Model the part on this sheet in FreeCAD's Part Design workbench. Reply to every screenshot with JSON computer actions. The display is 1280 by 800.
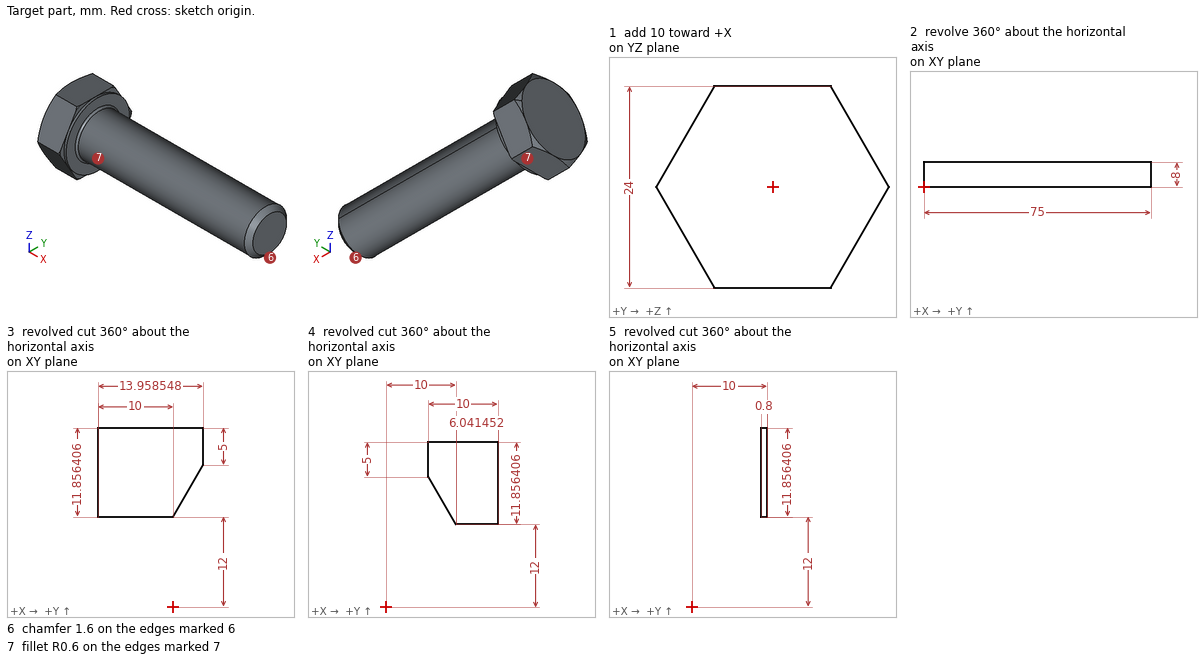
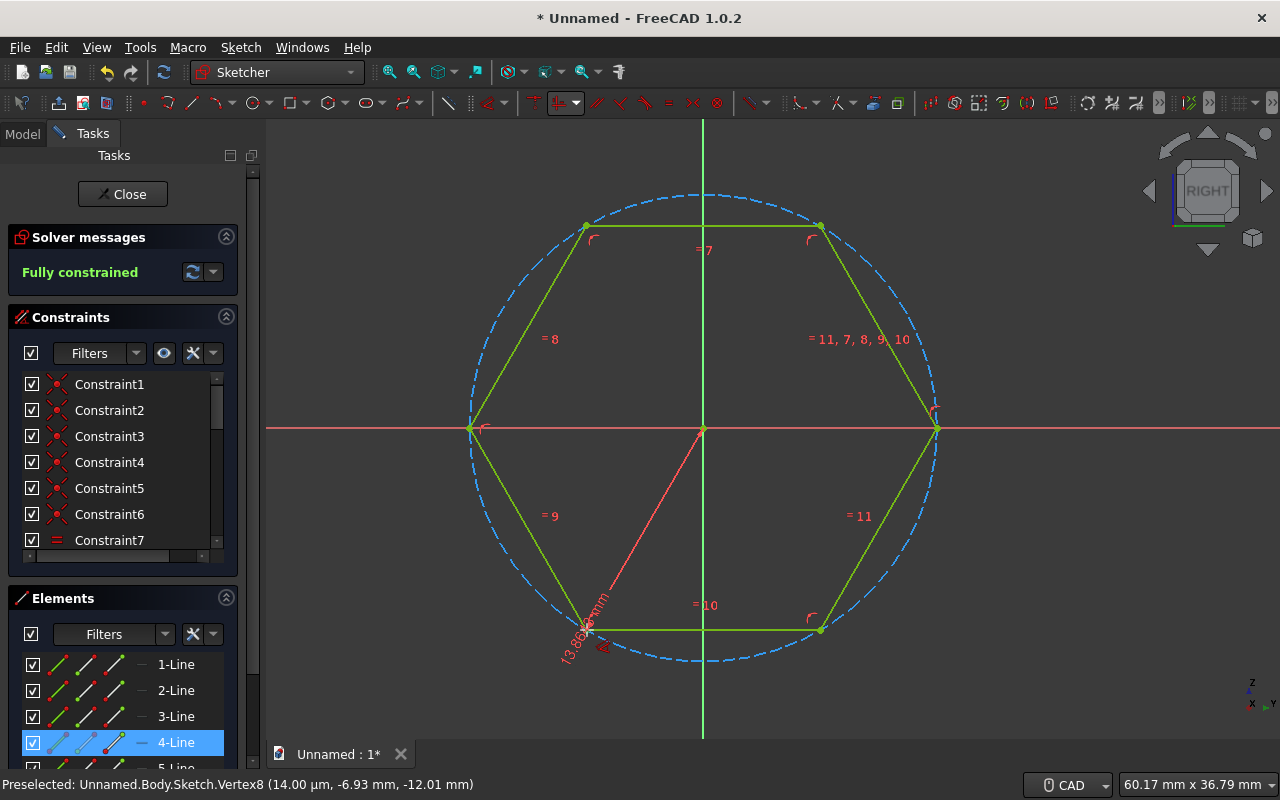
{"action": "left_click", "coordinate": [820, 226]}
{"action": "left_click", "coordinate": [553, 335]}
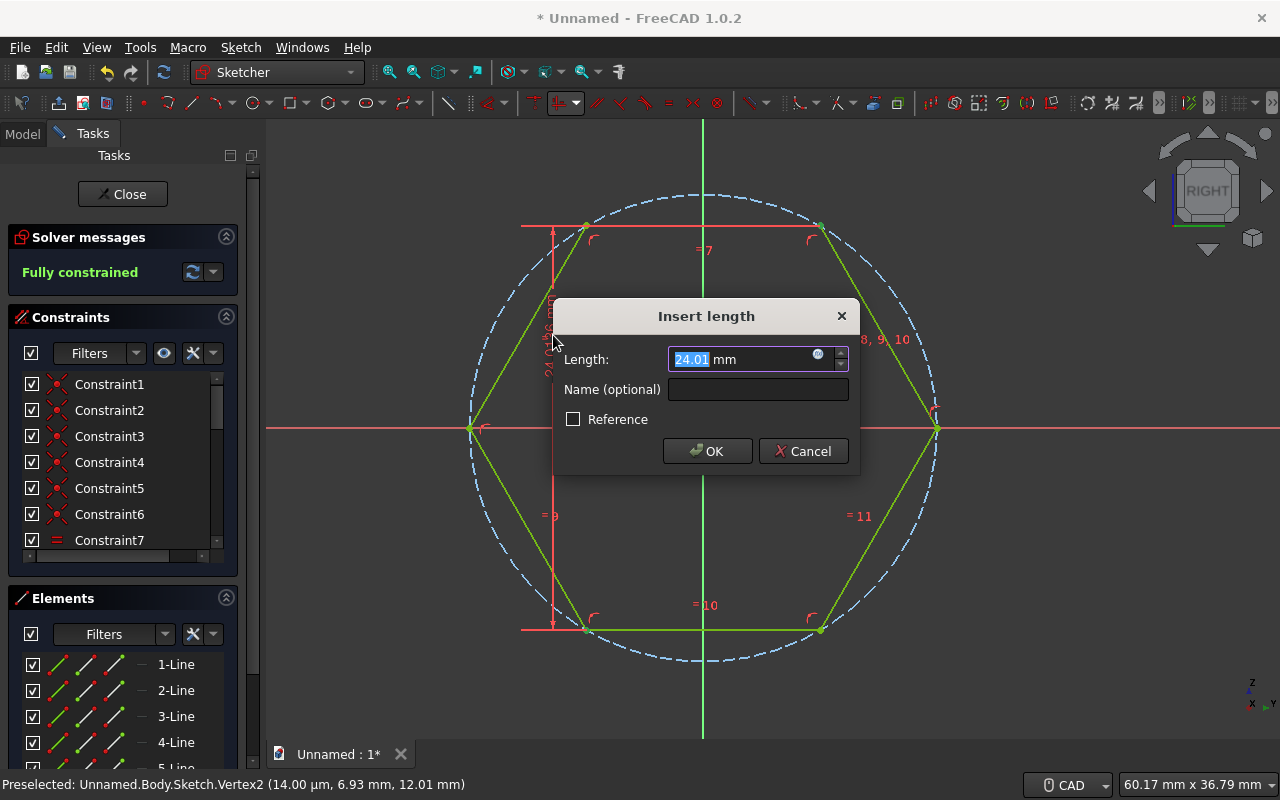
{"action": "type", "text": "24"}
{"action": "key", "text": "Return"}
{"action": "key", "text": "Escape"}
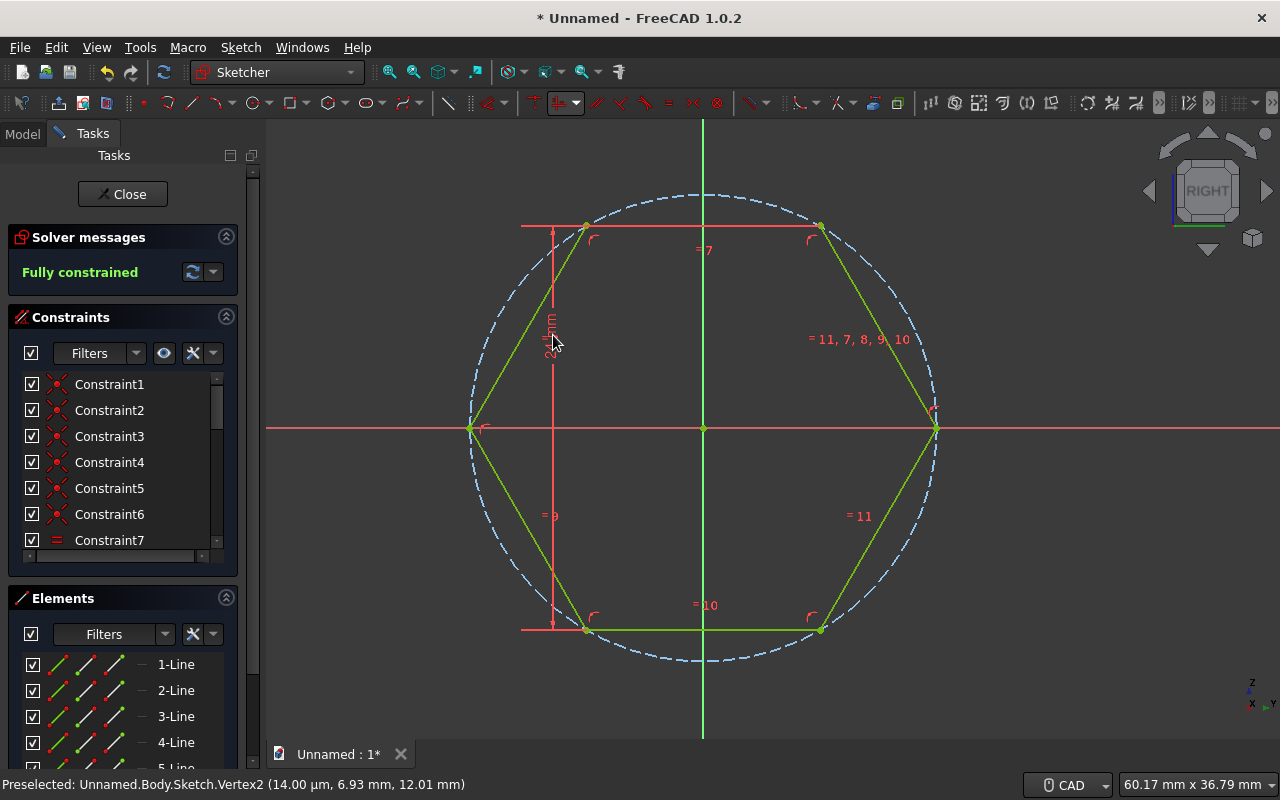
{"action": "left_click", "coordinate": [123, 194]}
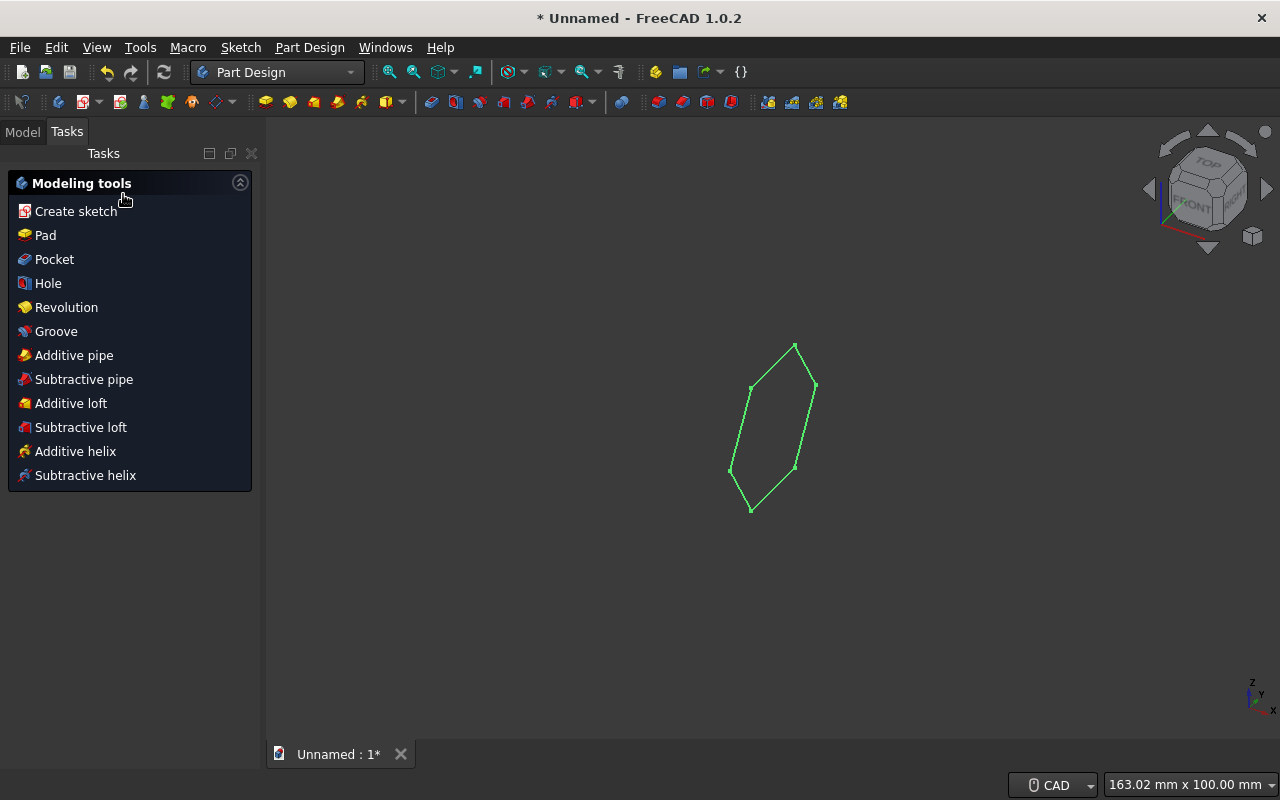
{"action": "left_click", "coordinate": [266, 102]}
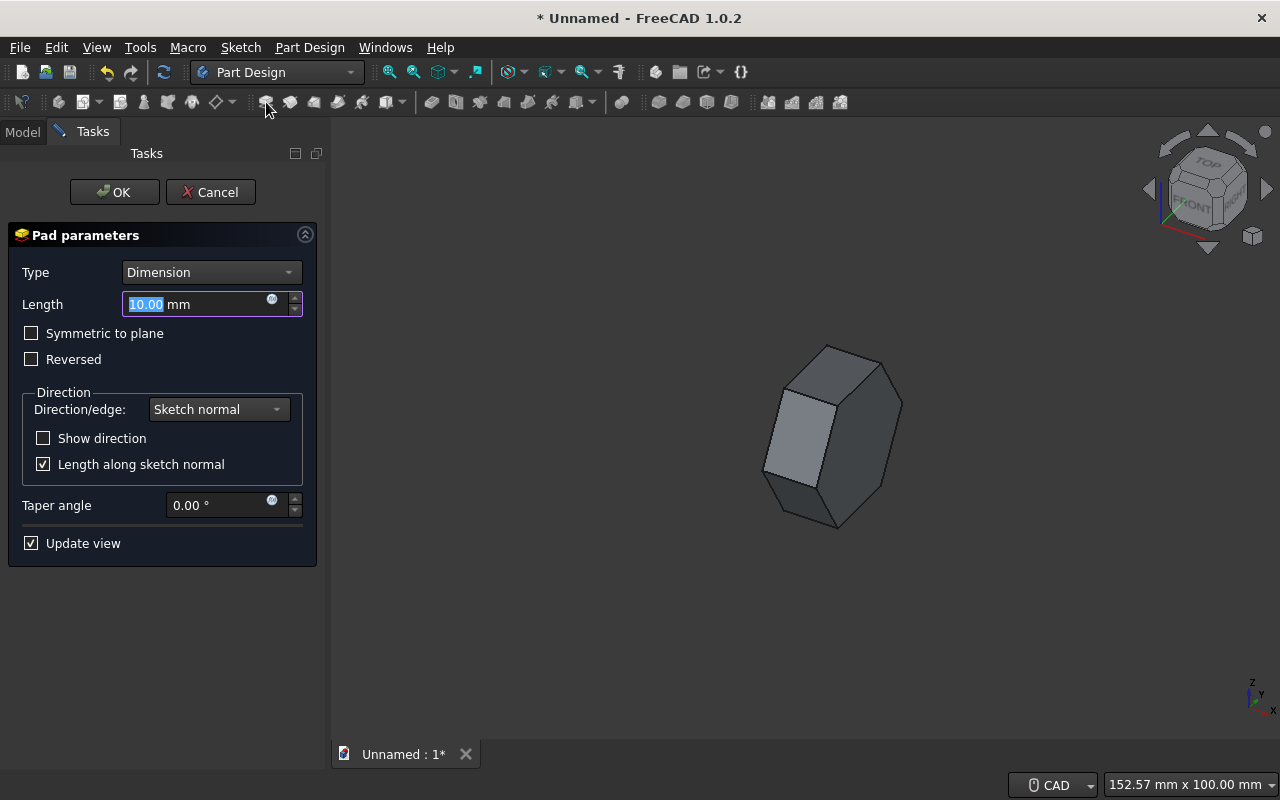
{"action": "type", "text": "10"}
{"action": "key", "text": "Tab"}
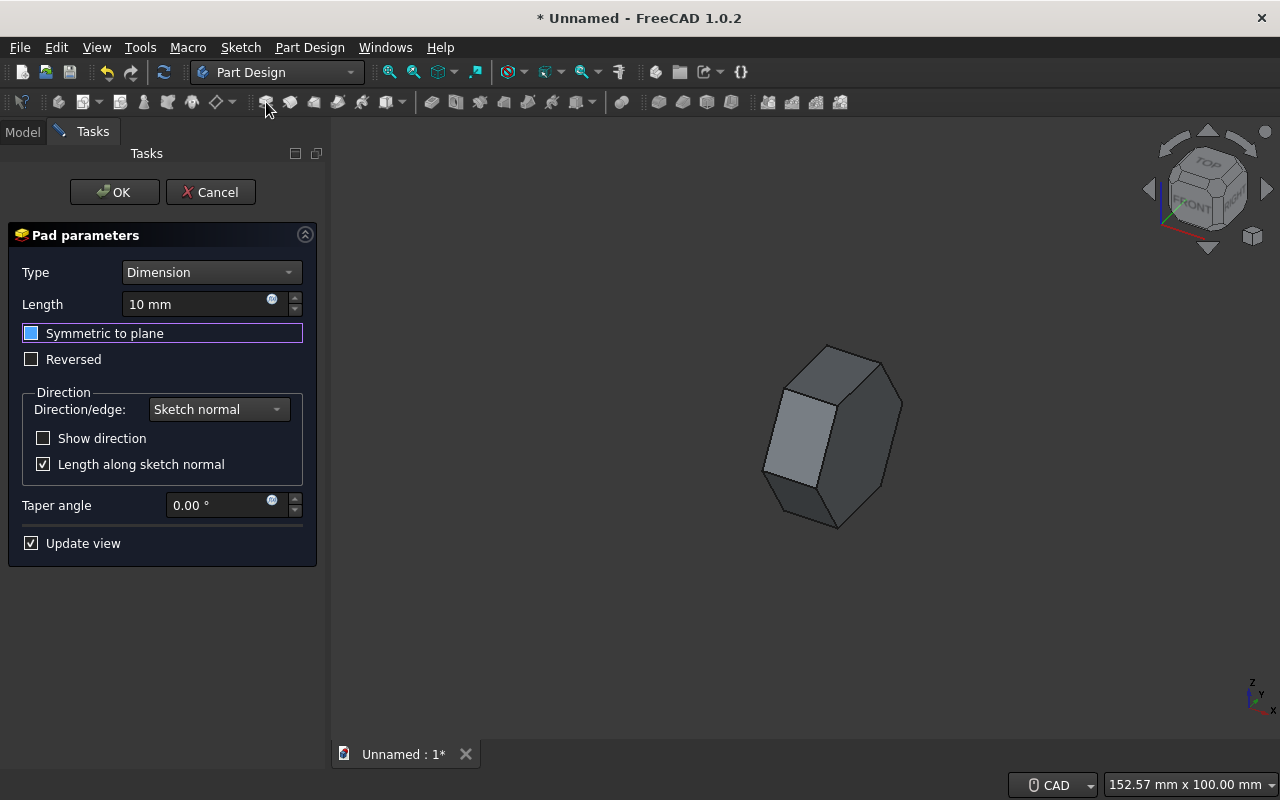
{"action": "left_click", "coordinate": [115, 192]}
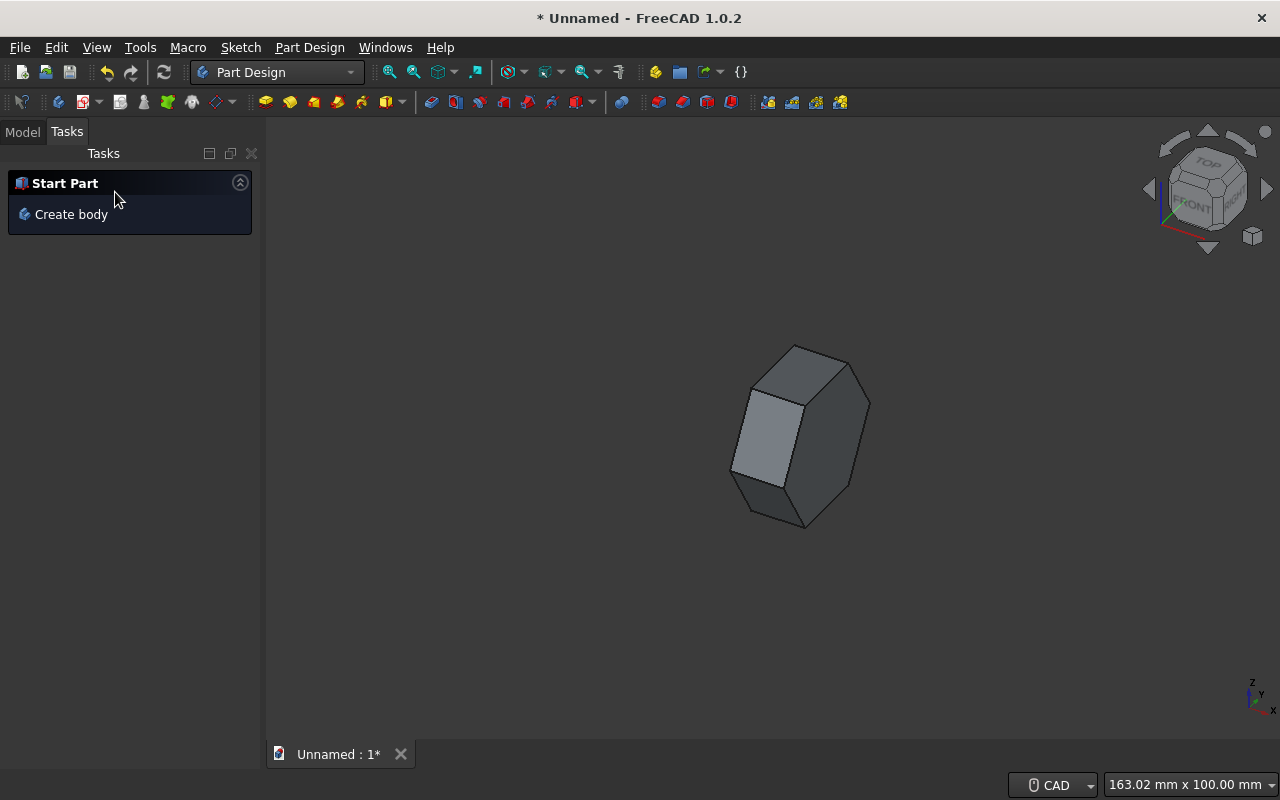
{"action": "left_click", "coordinate": [390, 72]}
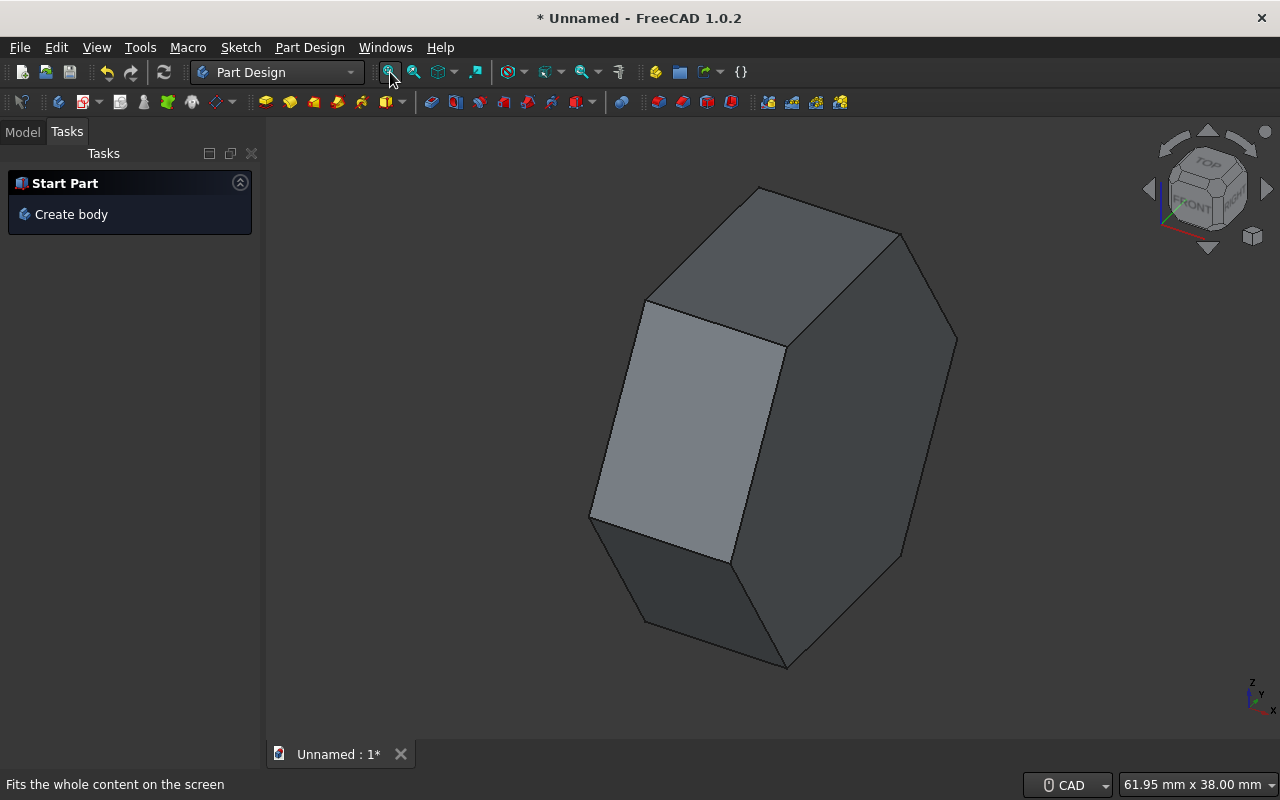
{"action": "left_click", "coordinate": [84, 102]}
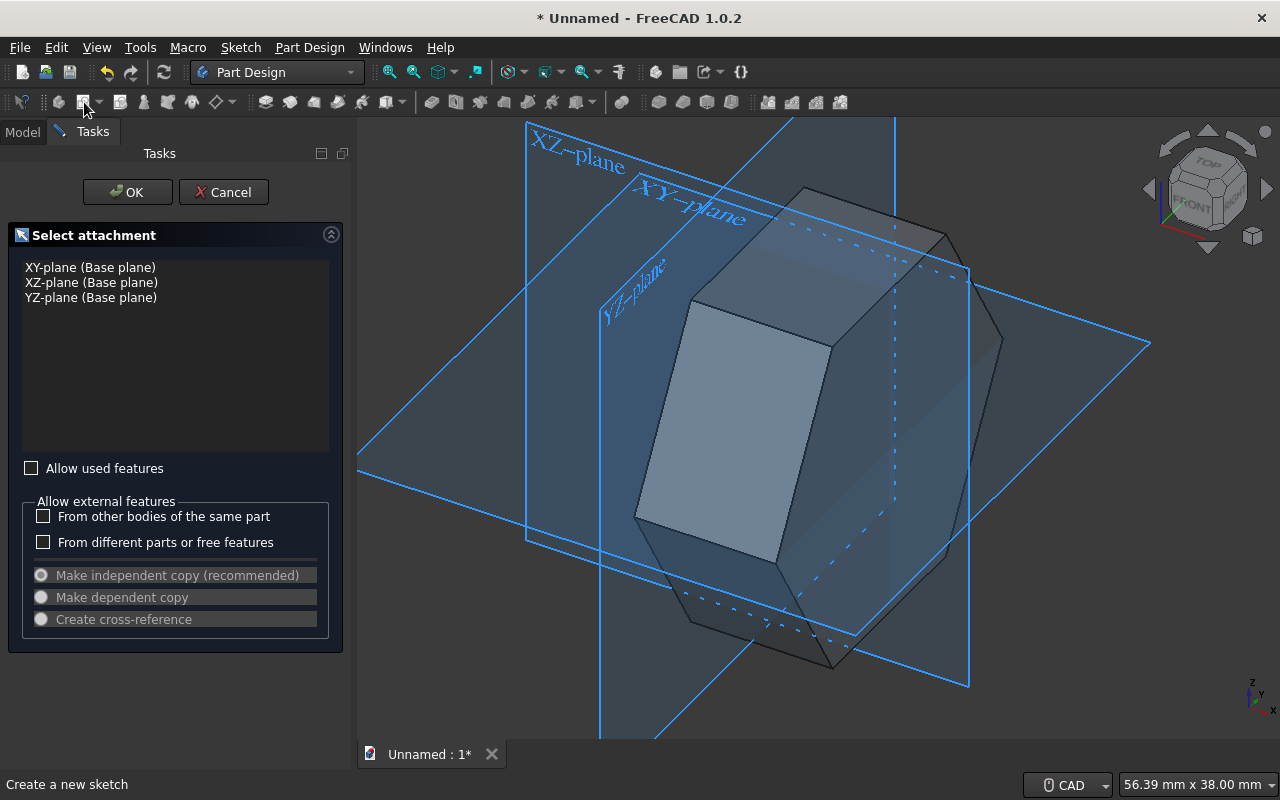
{"action": "left_click", "coordinate": [82, 268]}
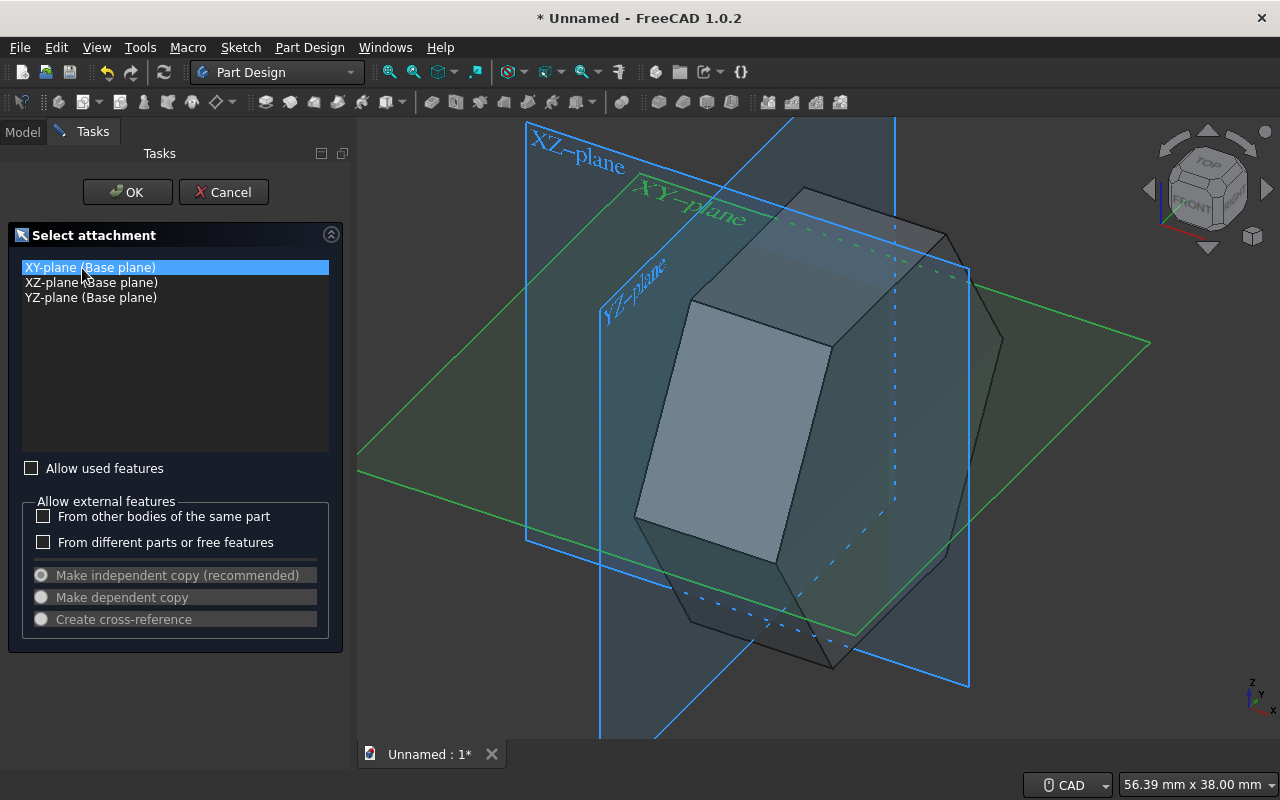
{"action": "left_click", "coordinate": [128, 192]}